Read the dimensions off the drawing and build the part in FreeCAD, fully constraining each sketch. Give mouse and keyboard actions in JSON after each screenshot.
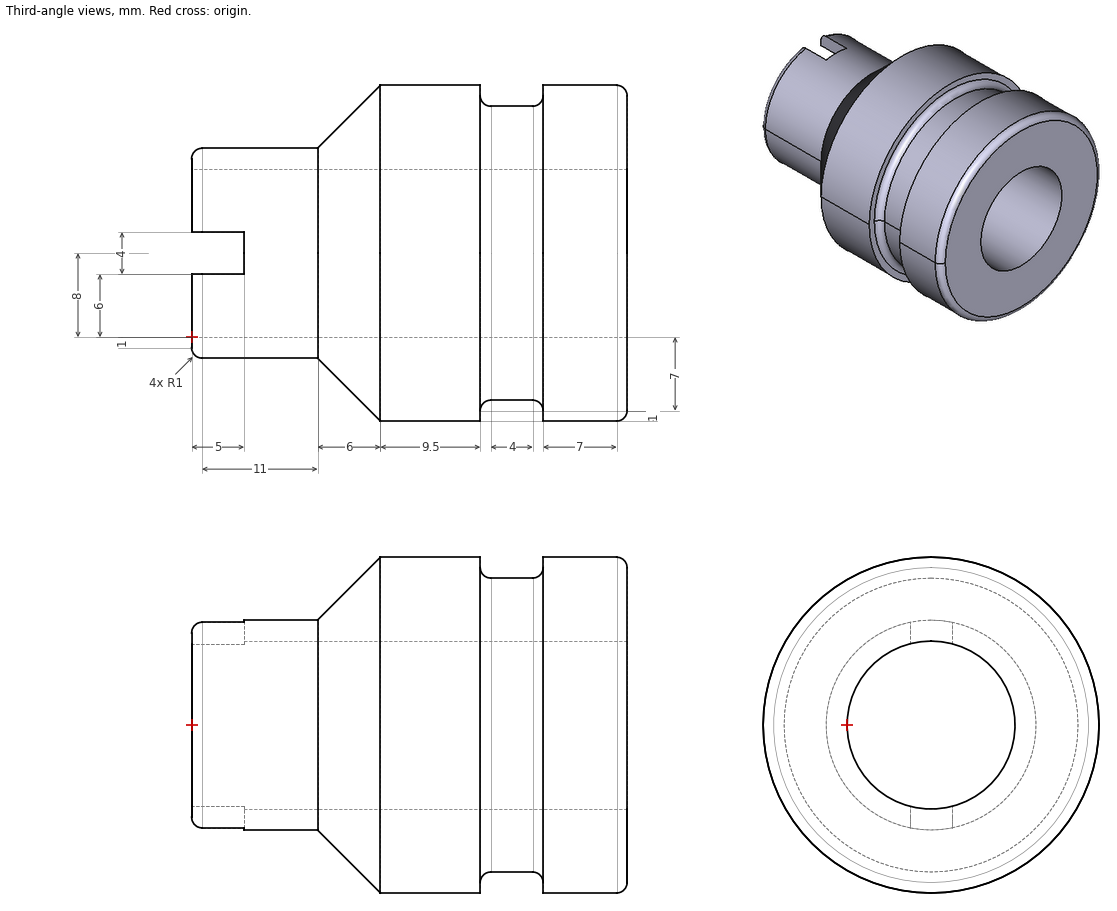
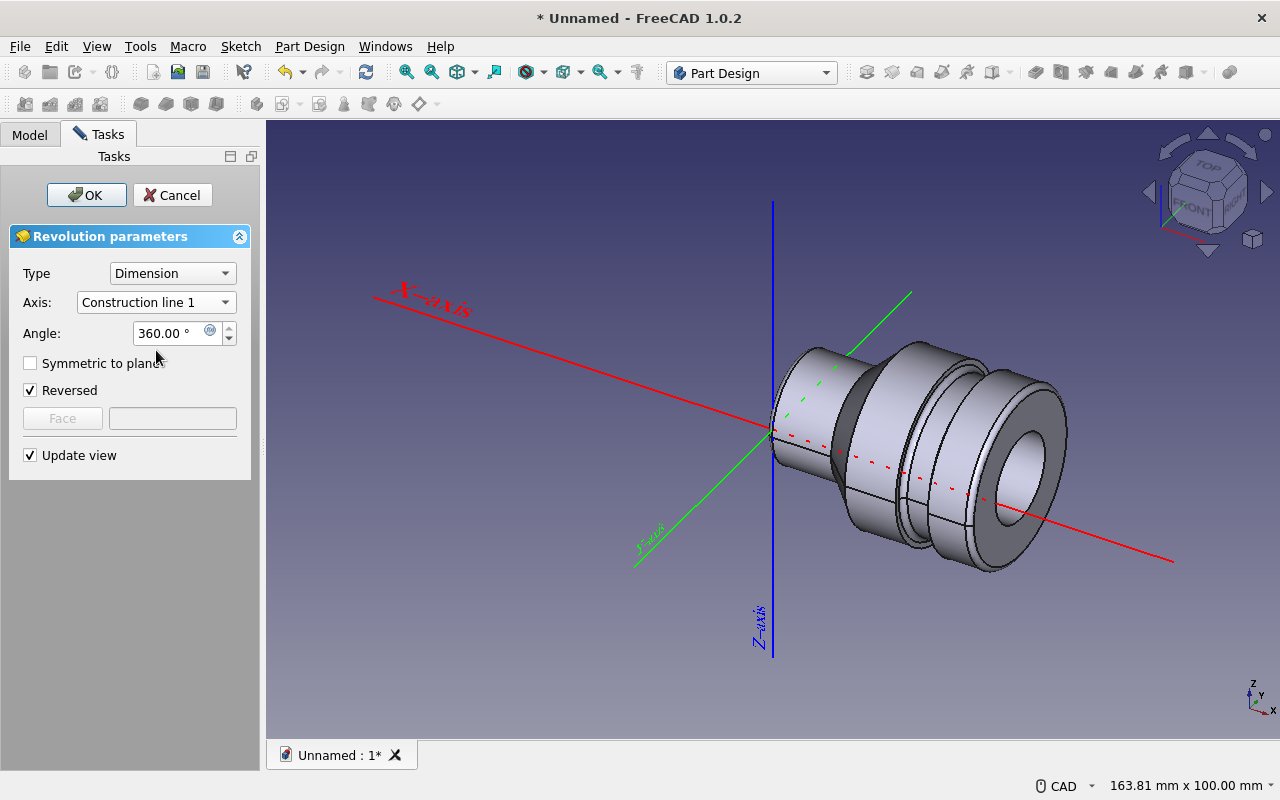
{"action": "left_click", "coordinate": [87, 195]}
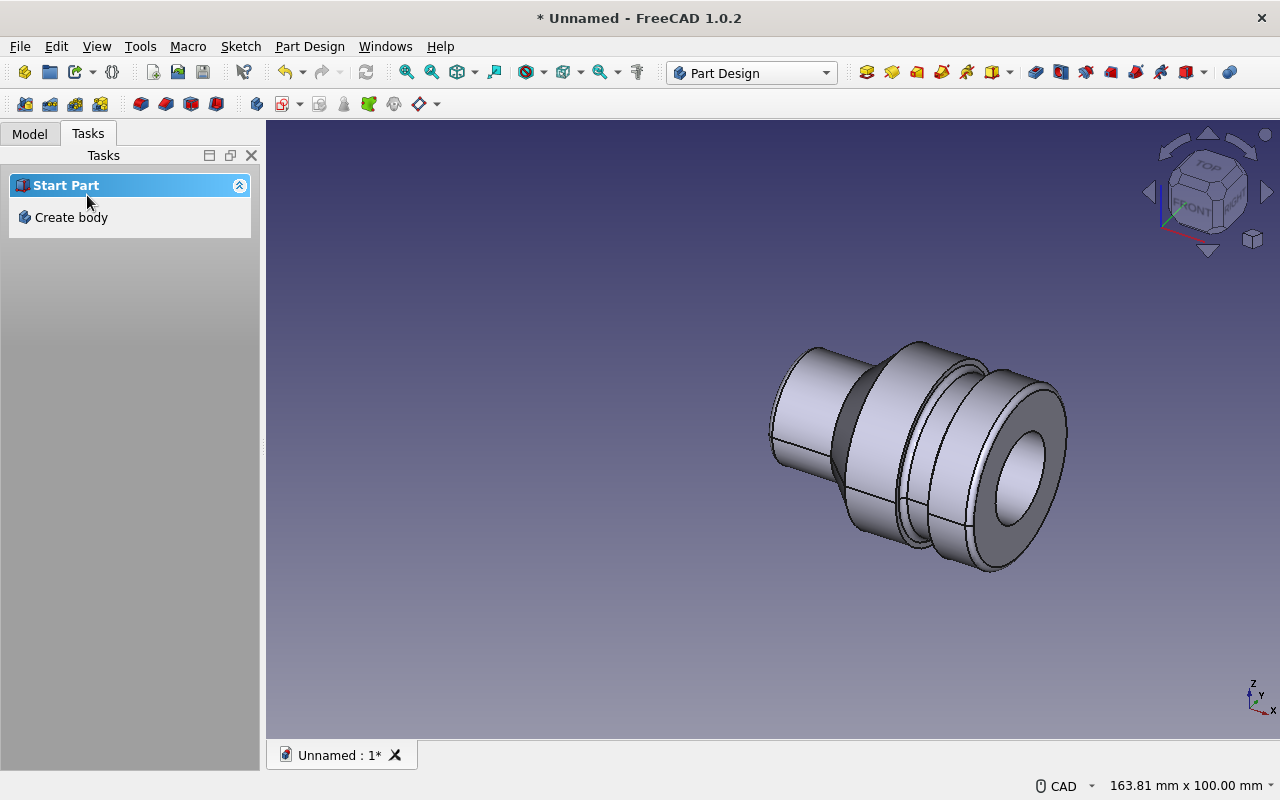
{"action": "left_click", "coordinate": [282, 104]}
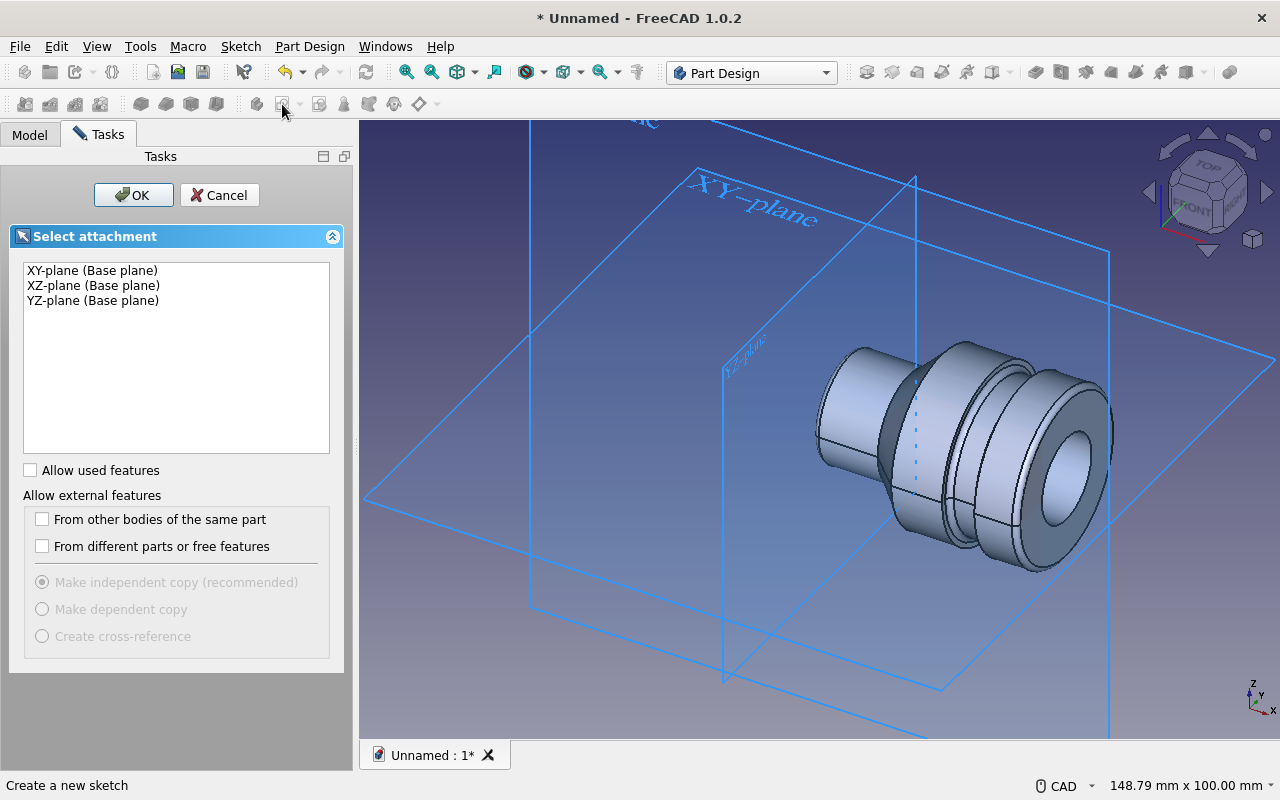
{"action": "left_click", "coordinate": [84, 270]}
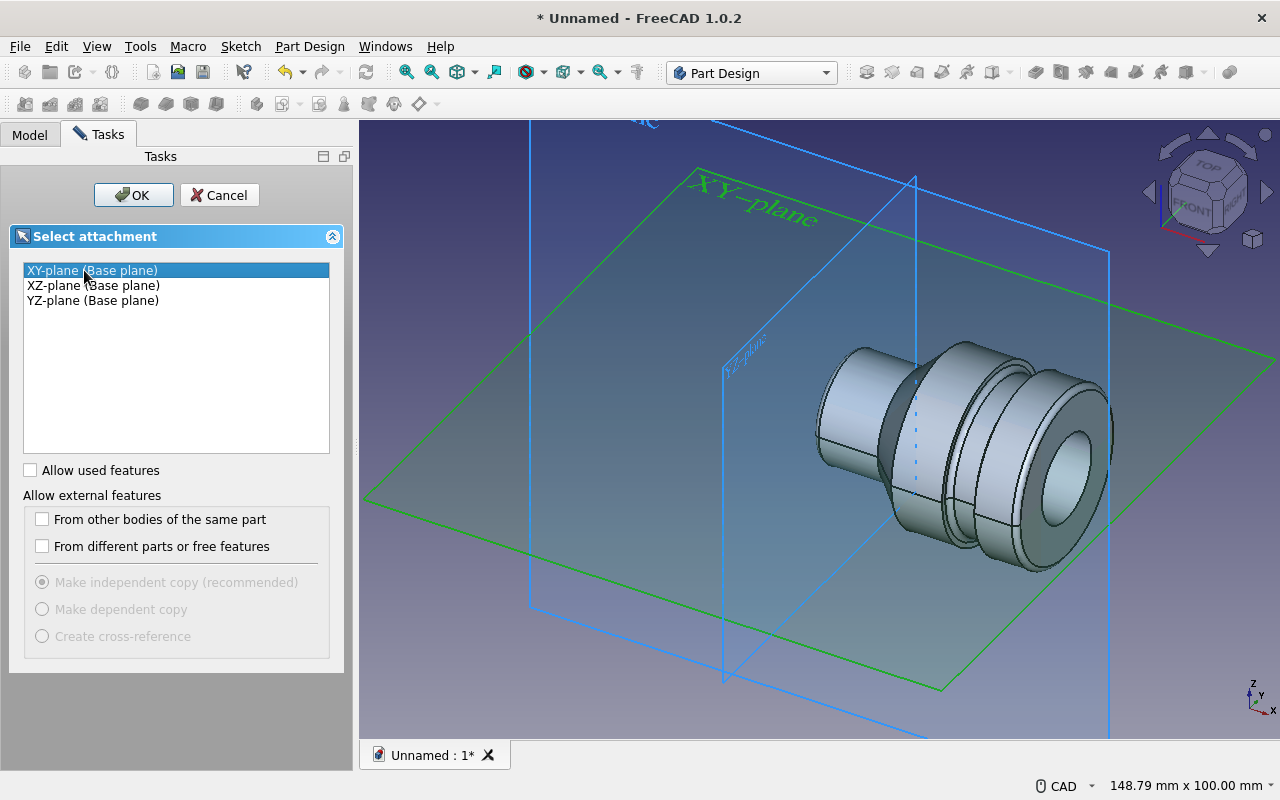
{"action": "left_click", "coordinate": [134, 195]}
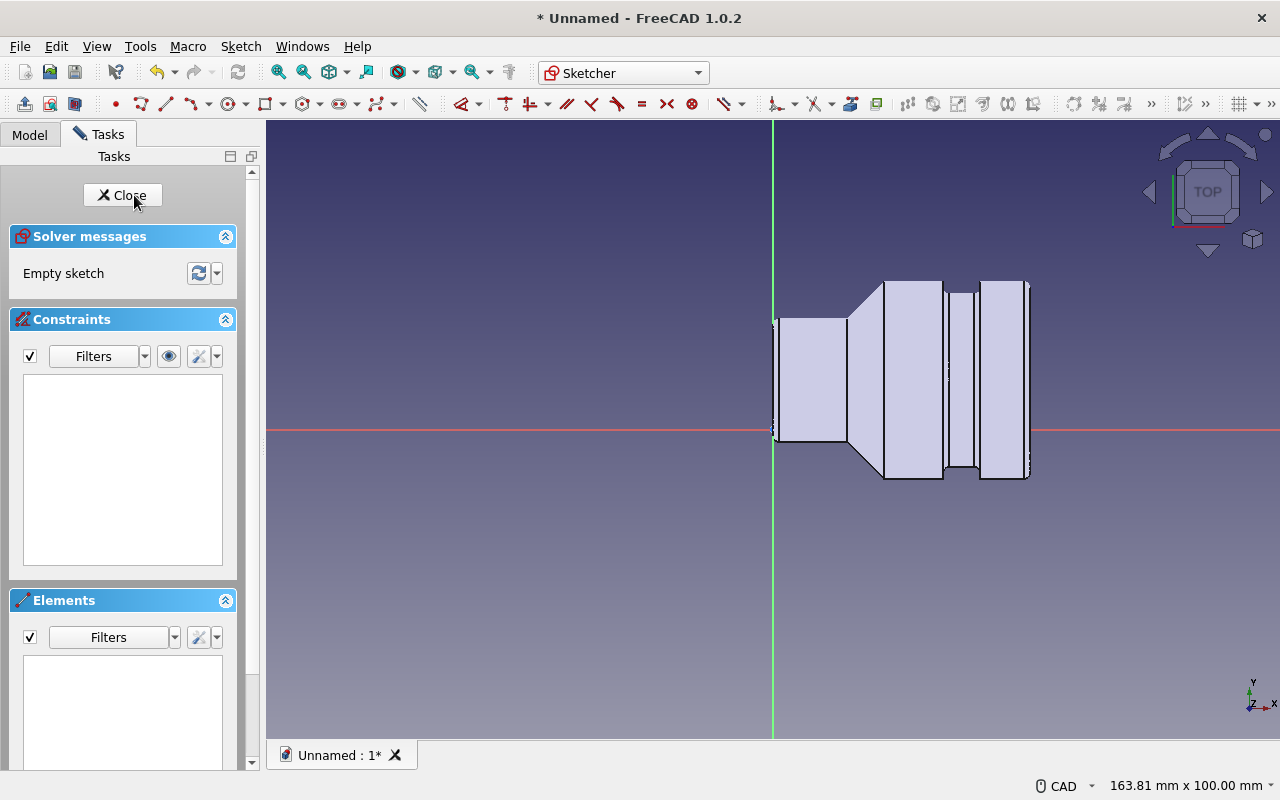
{"action": "key", "text": "q s"}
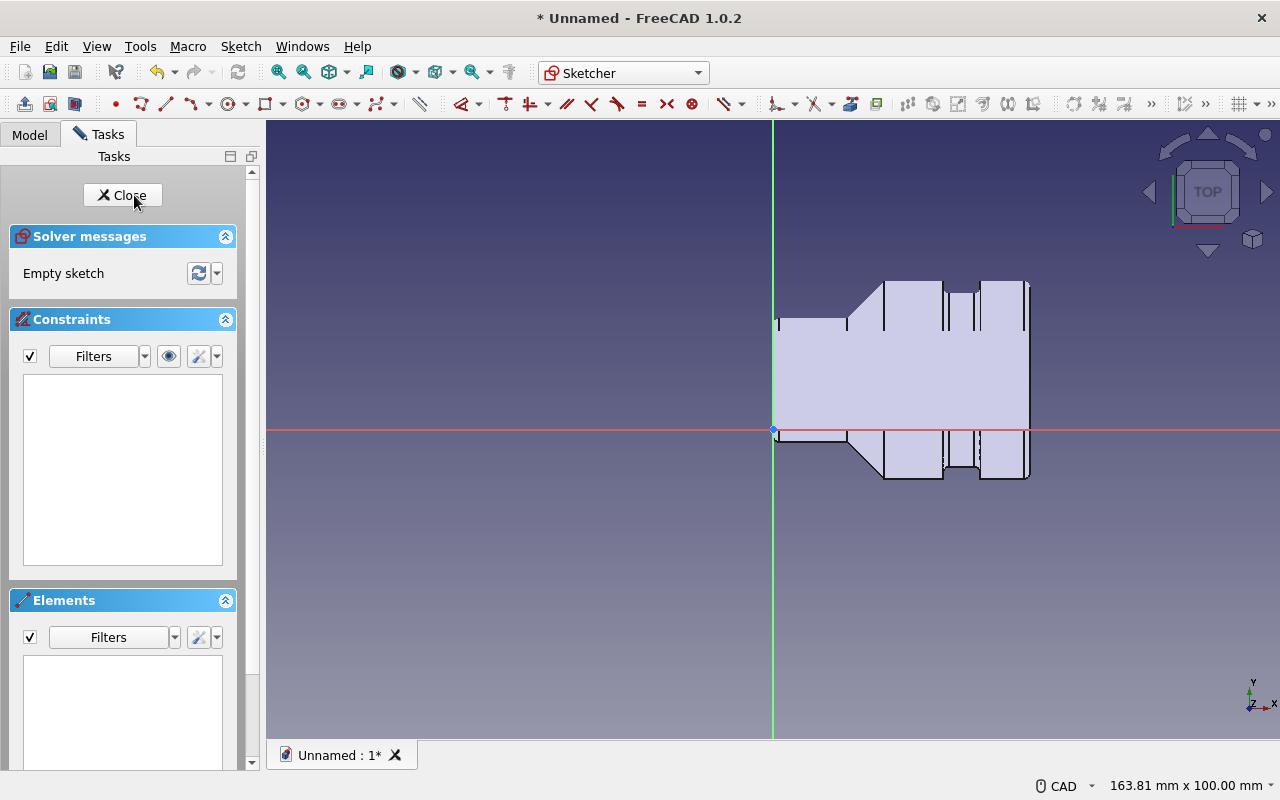
{"action": "scroll", "coordinate": [805, 392], "scroll_direction": "up", "scroll_amount": 9}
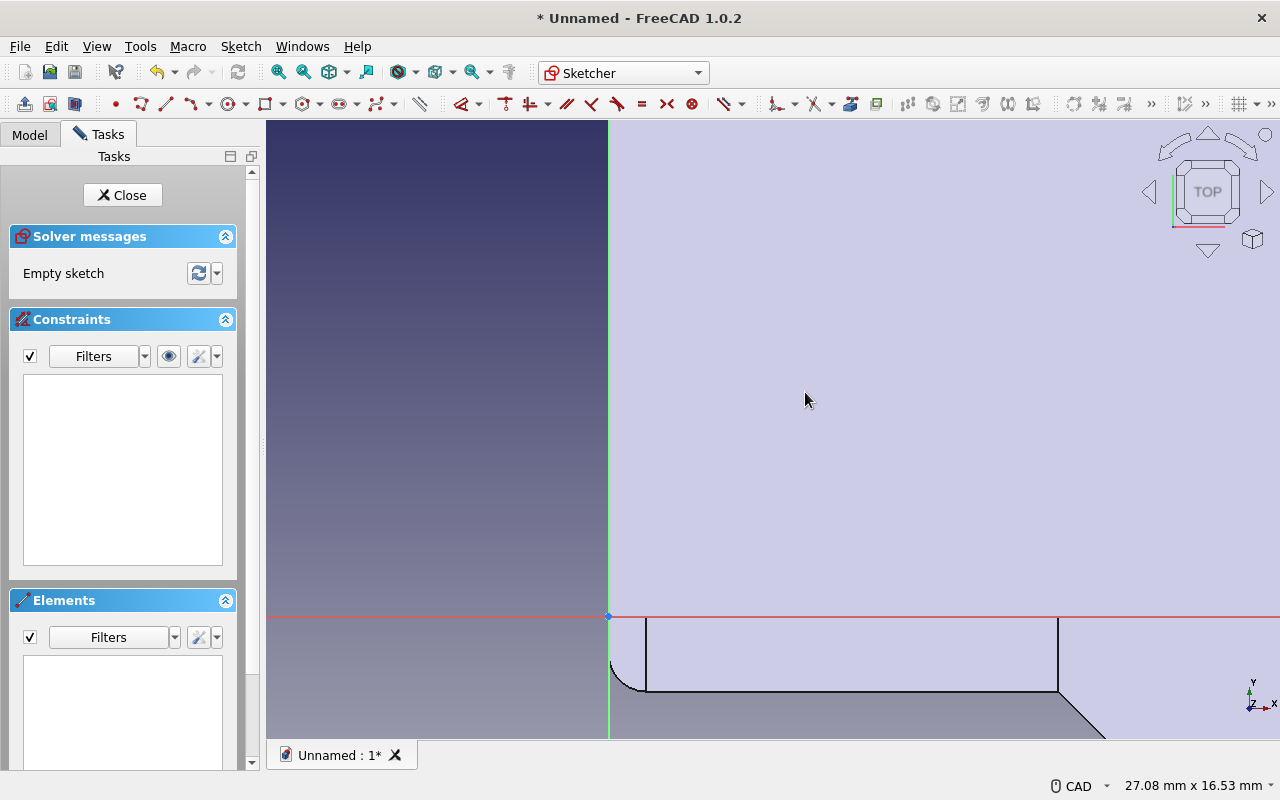
{"action": "key", "text": "g r"}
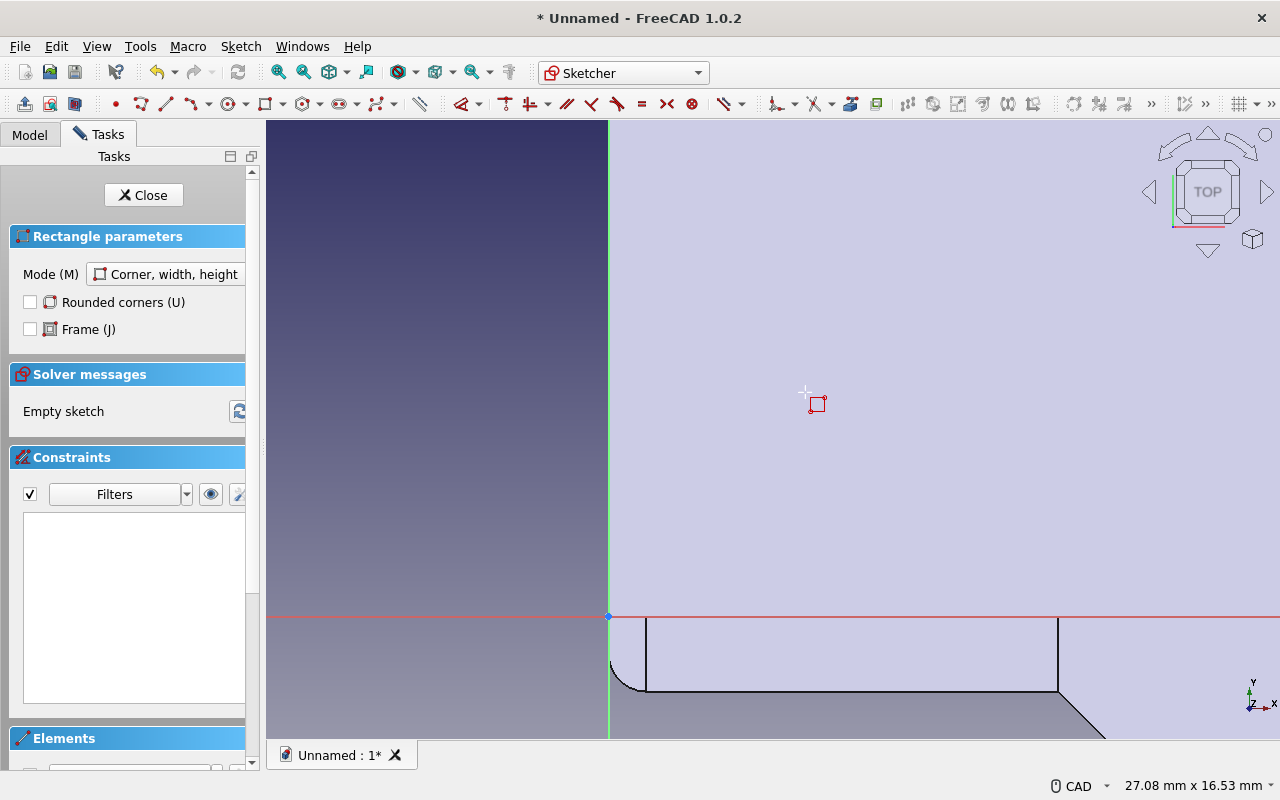
{"action": "left_click", "coordinate": [609, 242]}
{"action": "left_click", "coordinate": [796, 392]}
{"action": "key", "text": "Escape"}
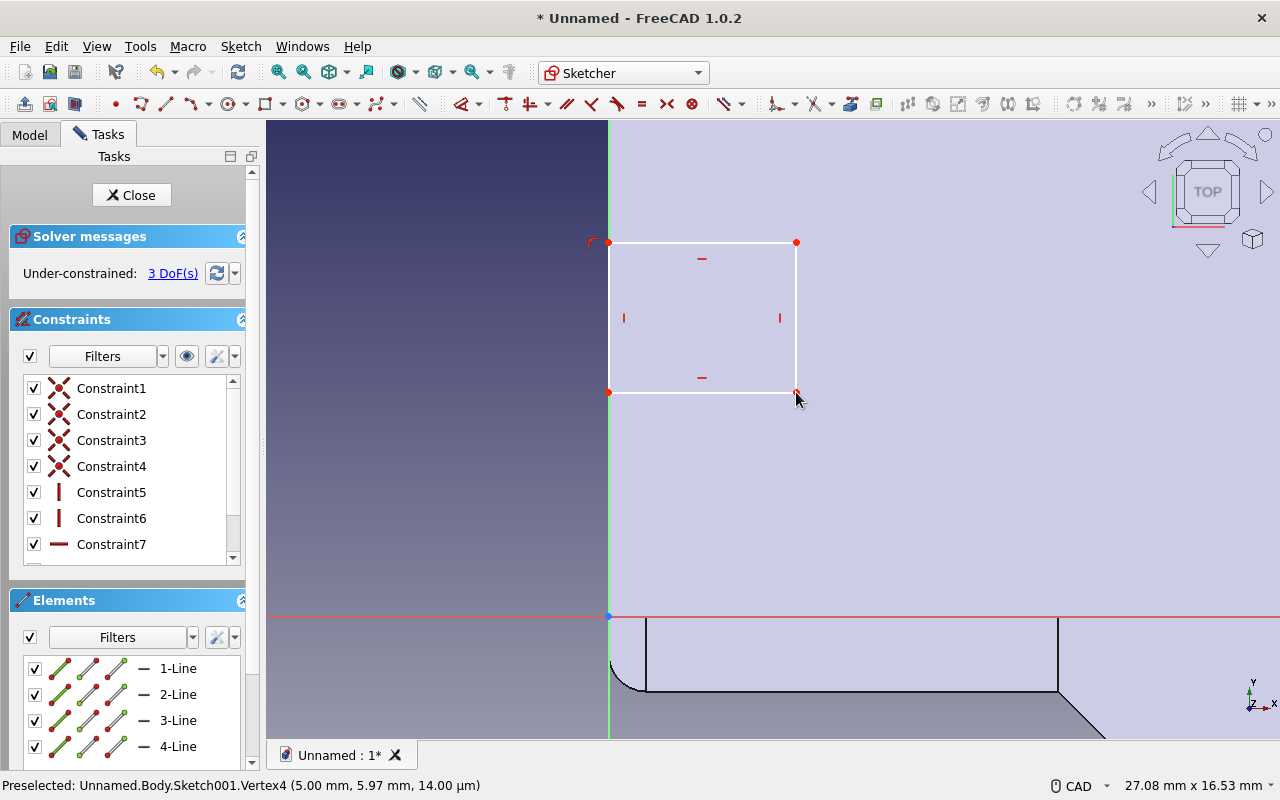
{"action": "left_click", "coordinate": [460, 104]}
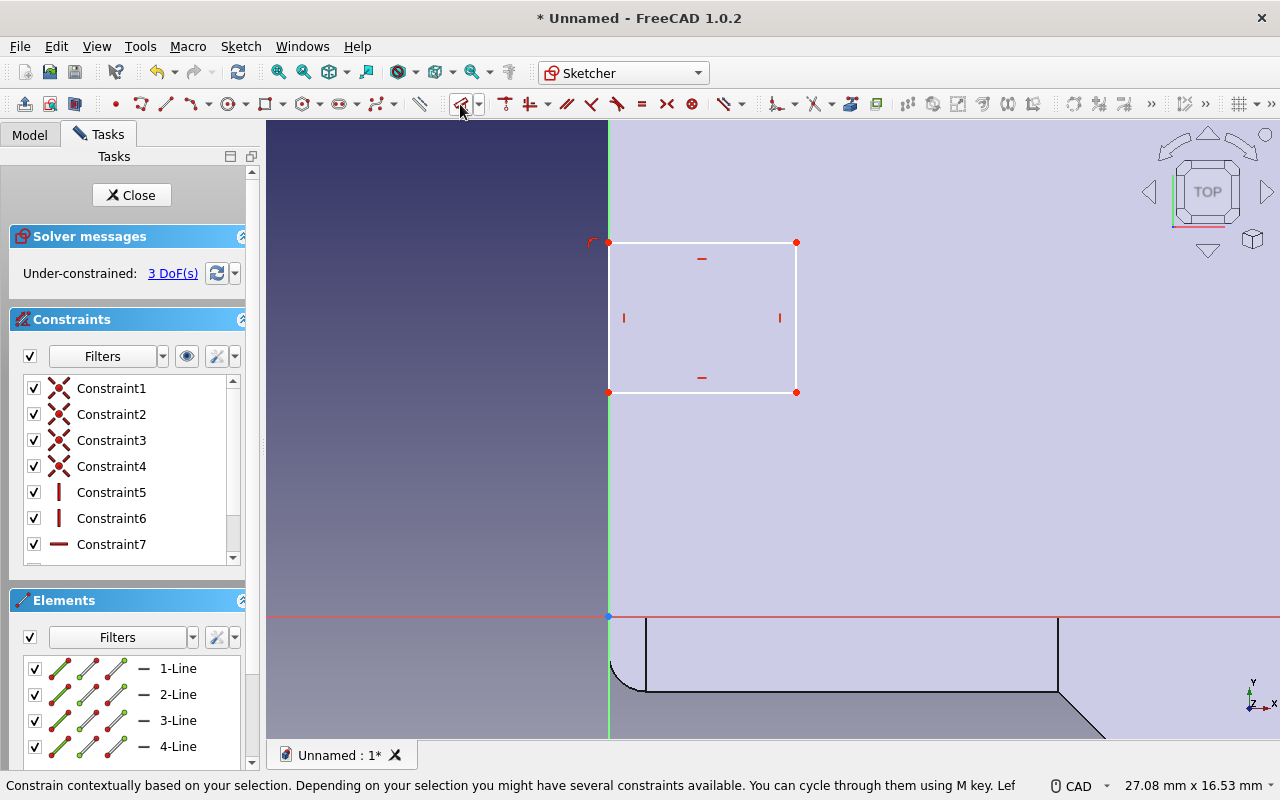
{"action": "left_click", "coordinate": [609, 288]}
{"action": "left_click", "coordinate": [575, 318]}